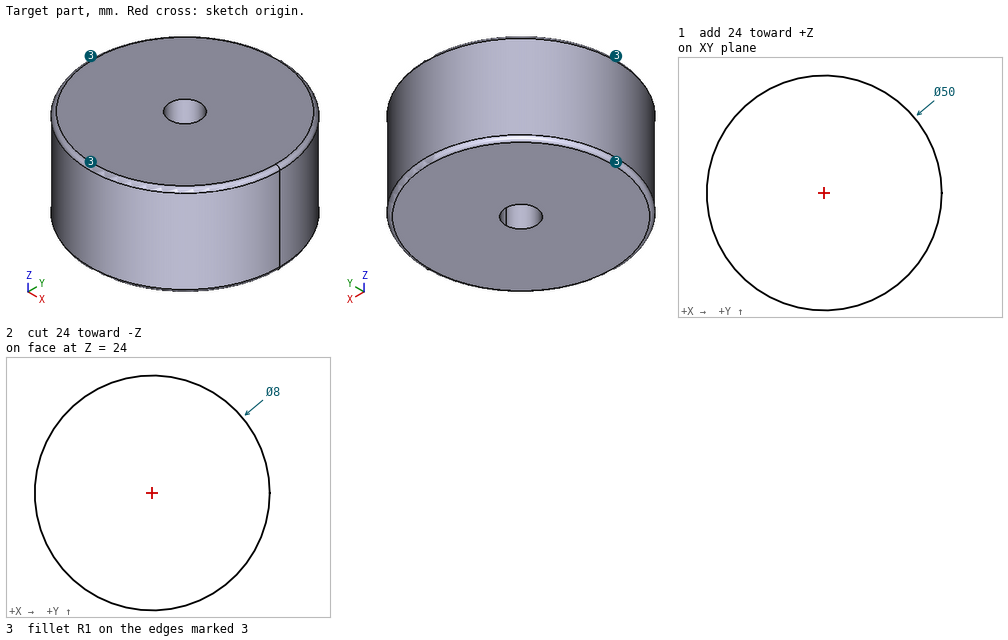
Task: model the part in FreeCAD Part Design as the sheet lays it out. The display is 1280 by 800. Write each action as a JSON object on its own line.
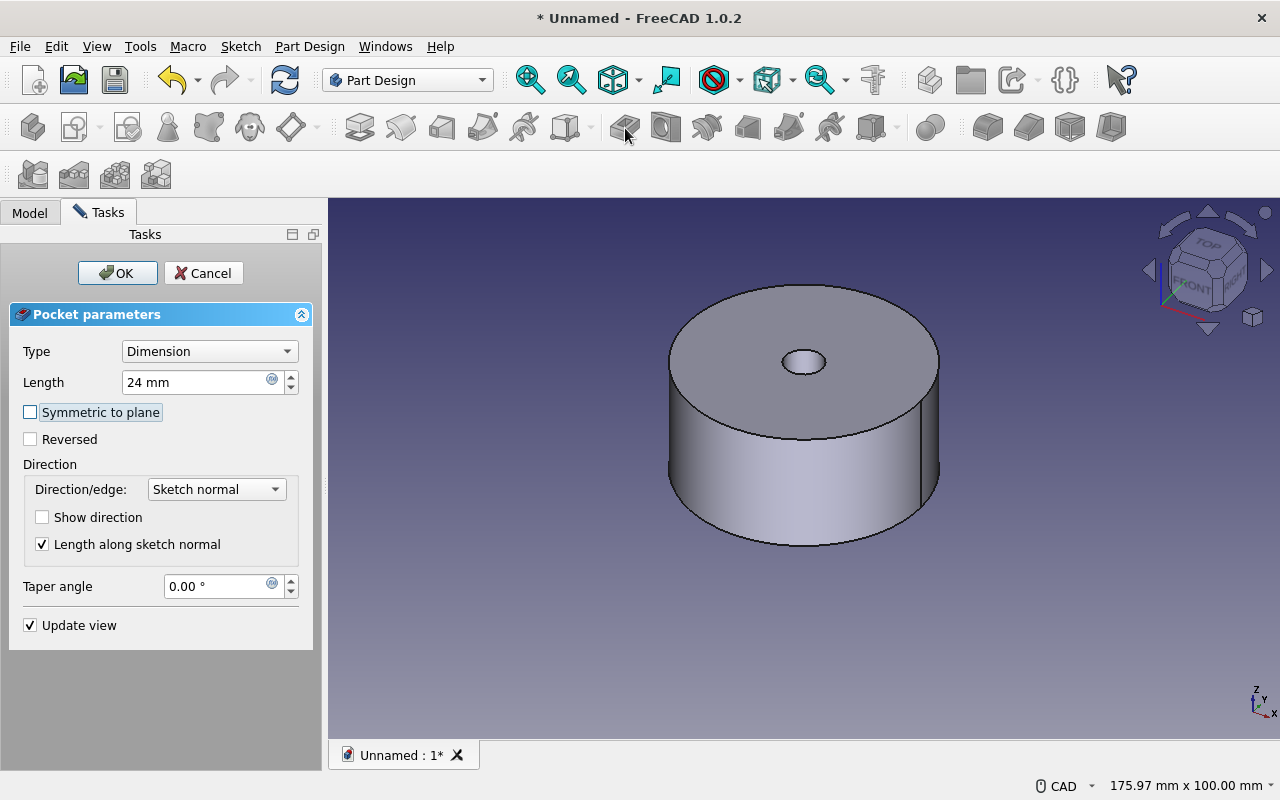
{"action": "left_click", "coordinate": [118, 273]}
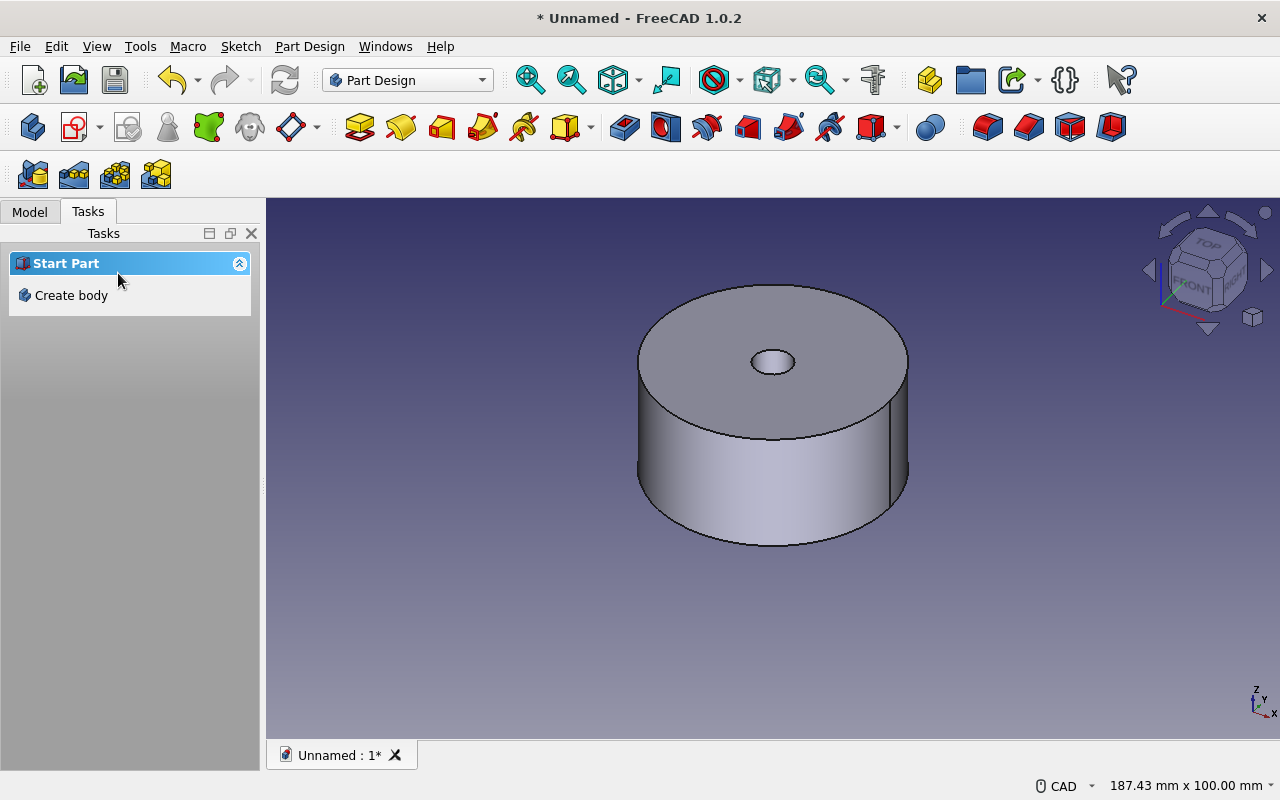
{"action": "left_click", "coordinate": [638, 369]}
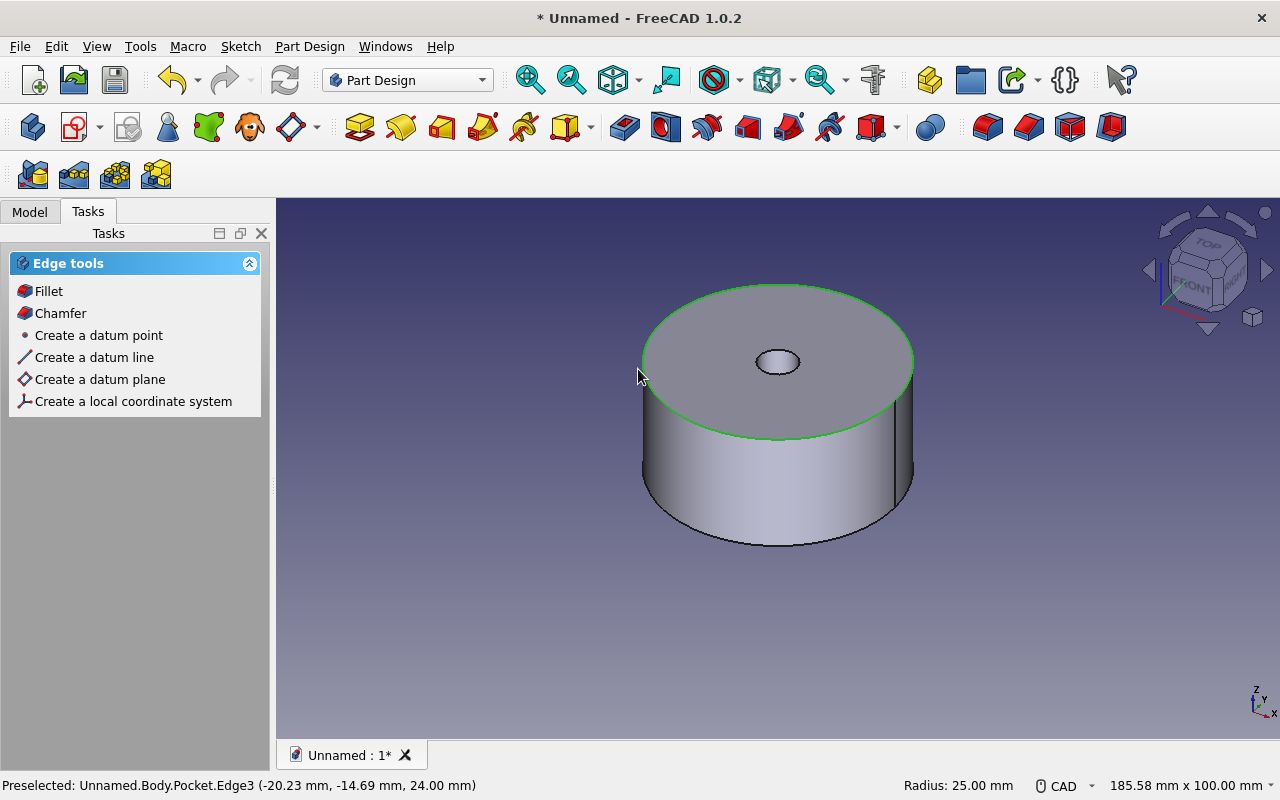
{"action": "key", "text": "0"}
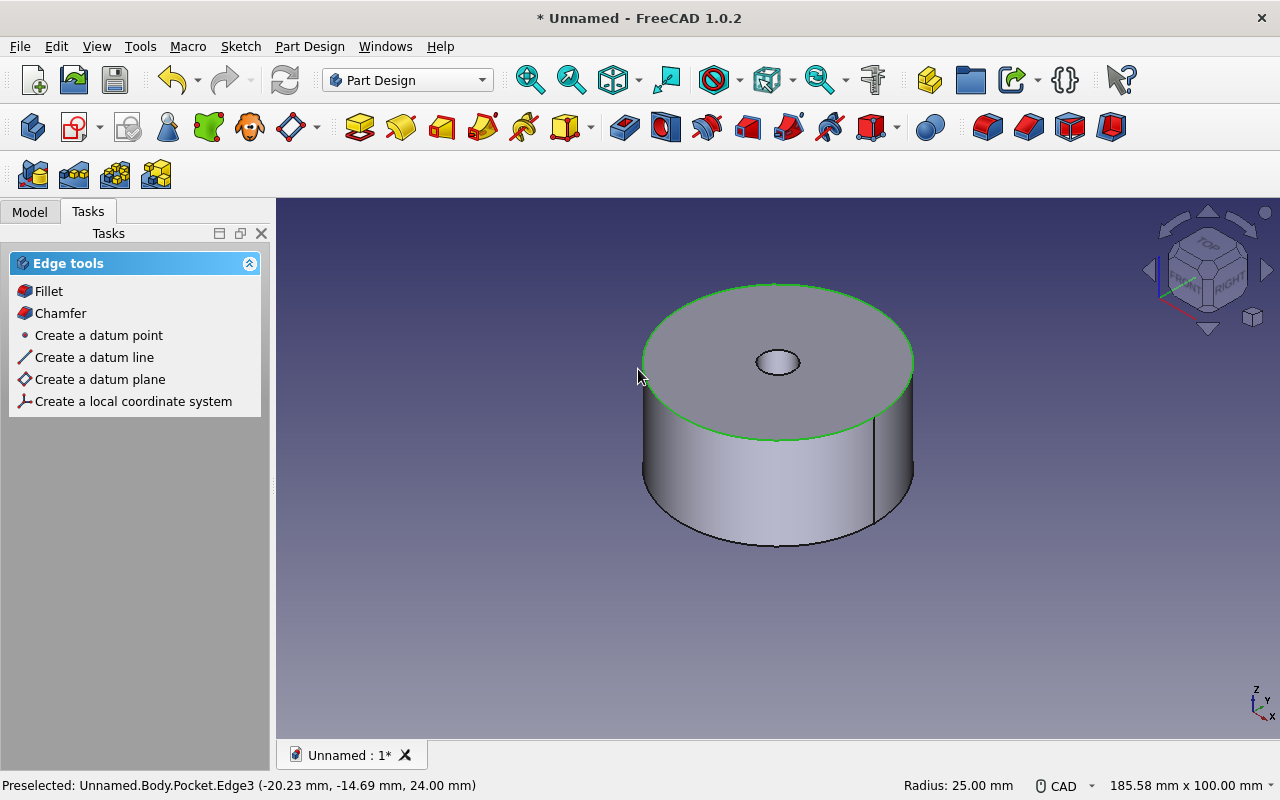
{"action": "key", "text": "2"}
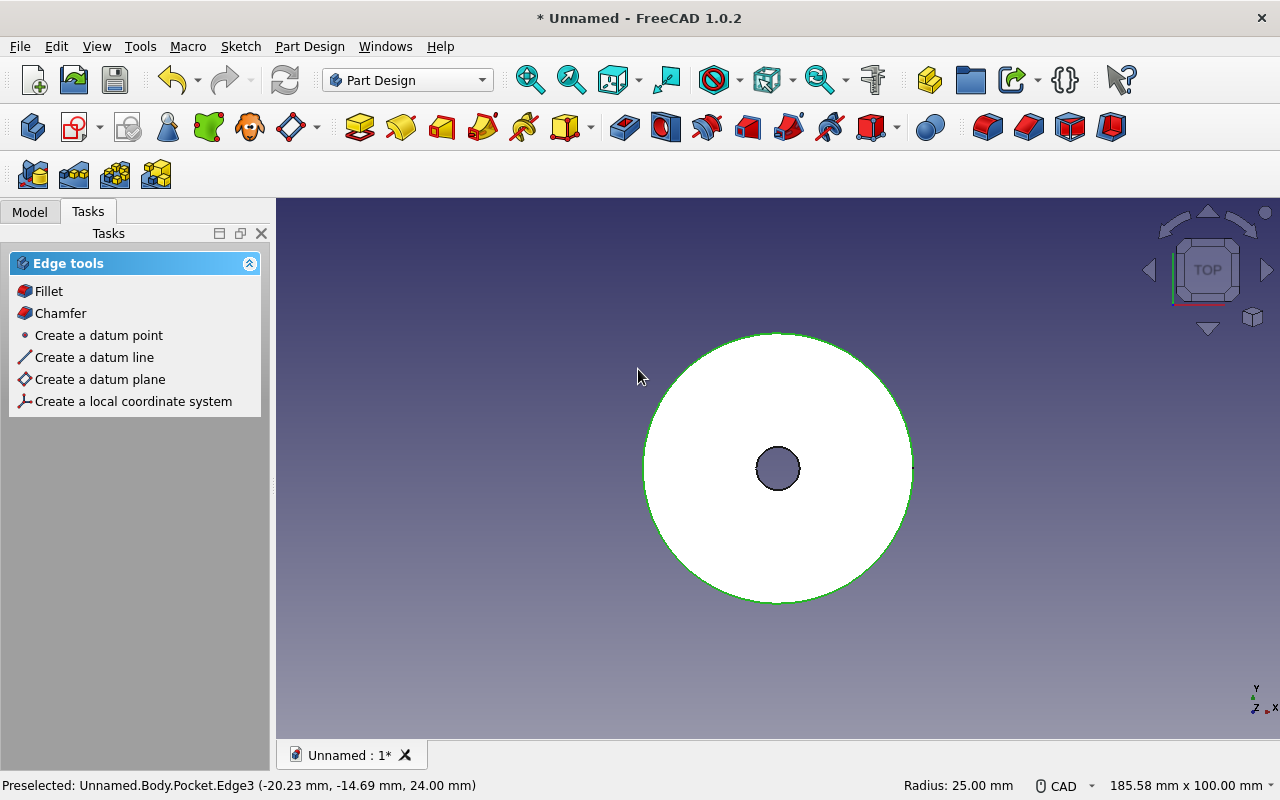
{"action": "key", "text": "1"}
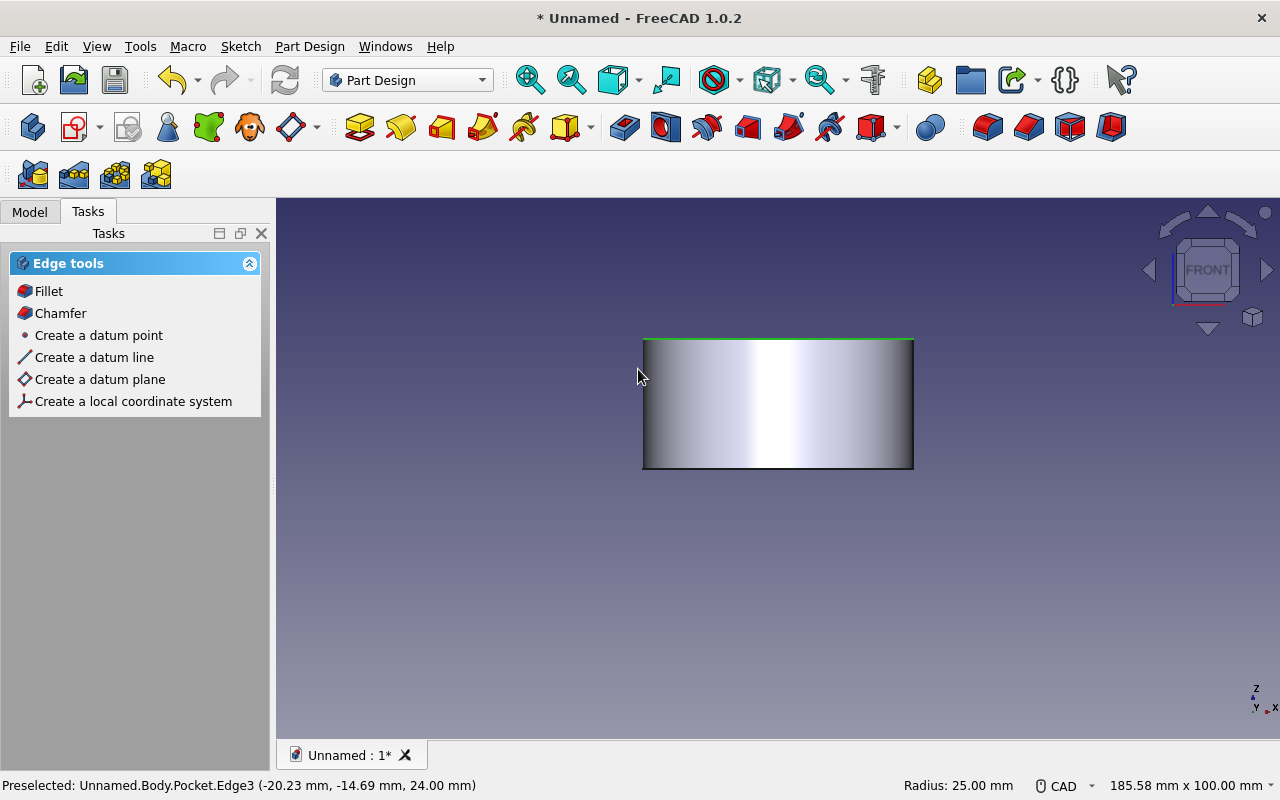
{"action": "left_click", "coordinate": [531, 80]}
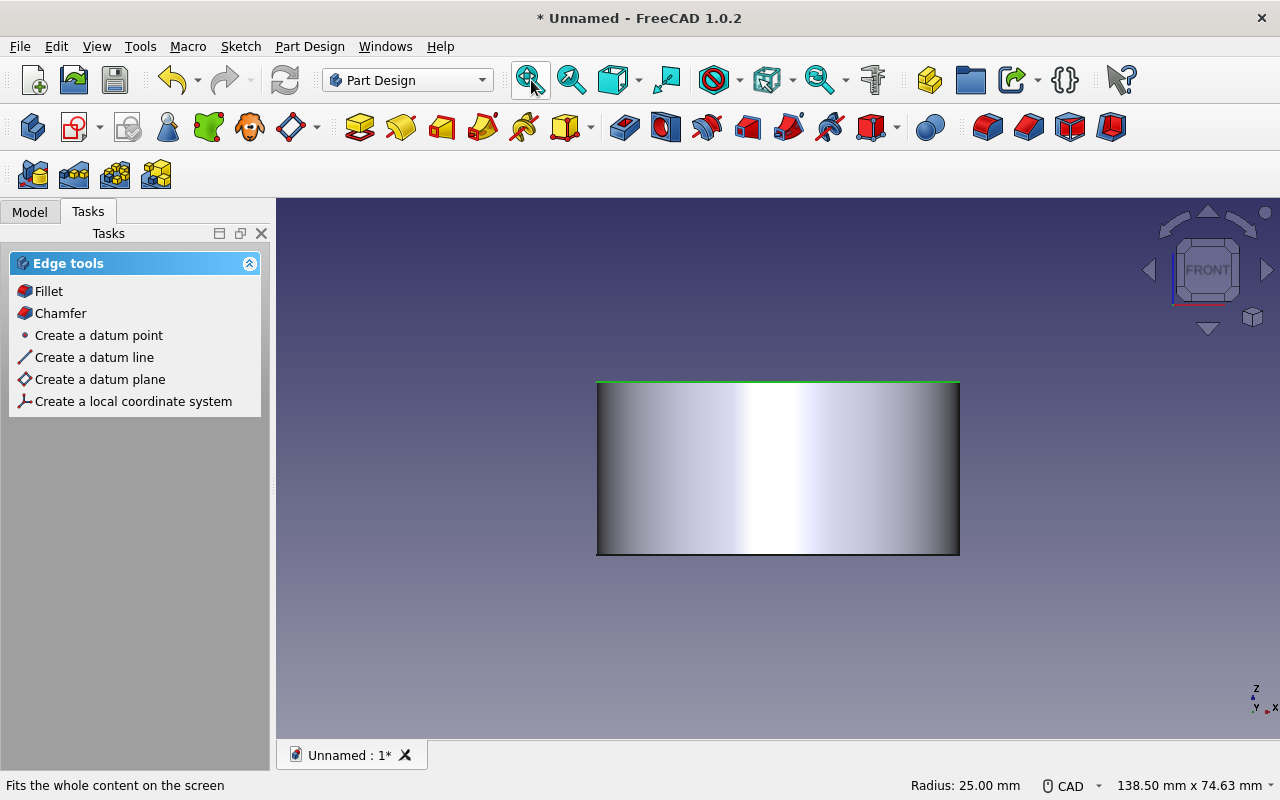
{"action": "left_click", "coordinate": [631, 554], "text": "ctrl"}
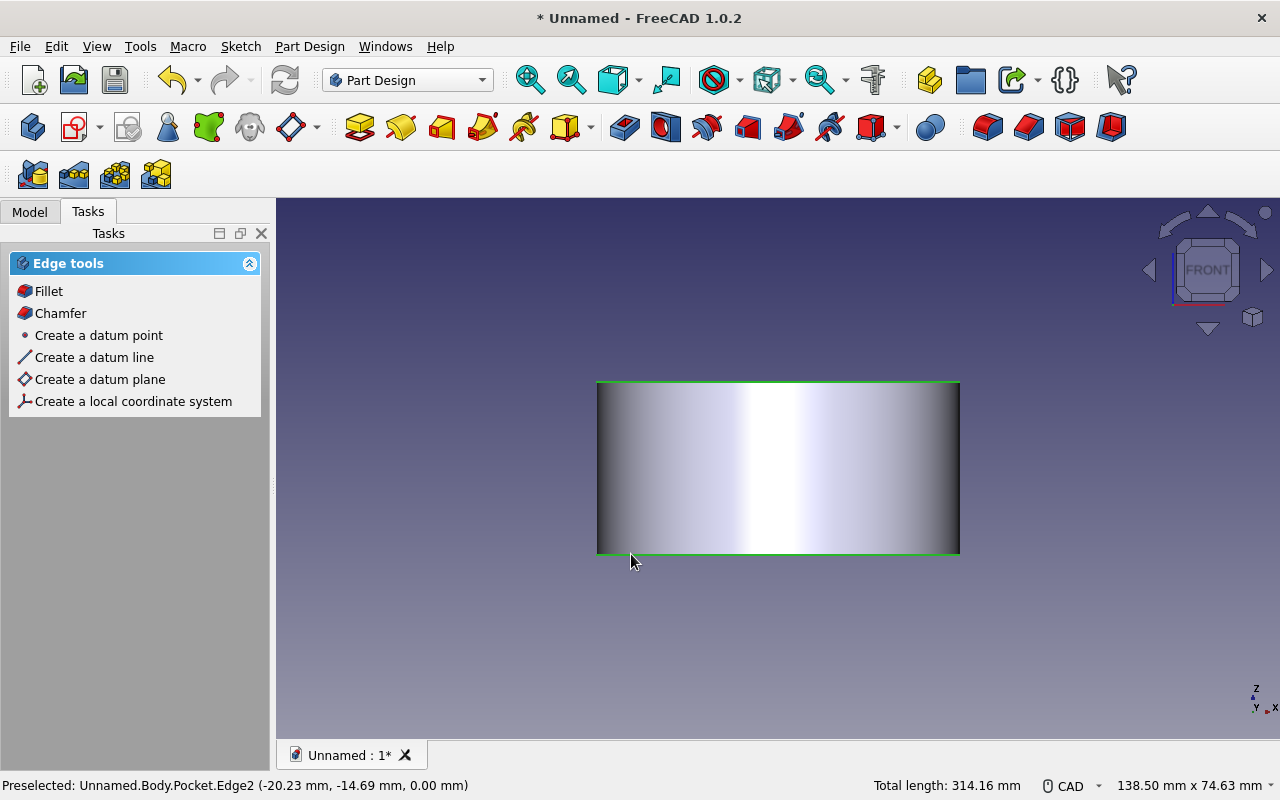
{"action": "left_click", "coordinate": [988, 128]}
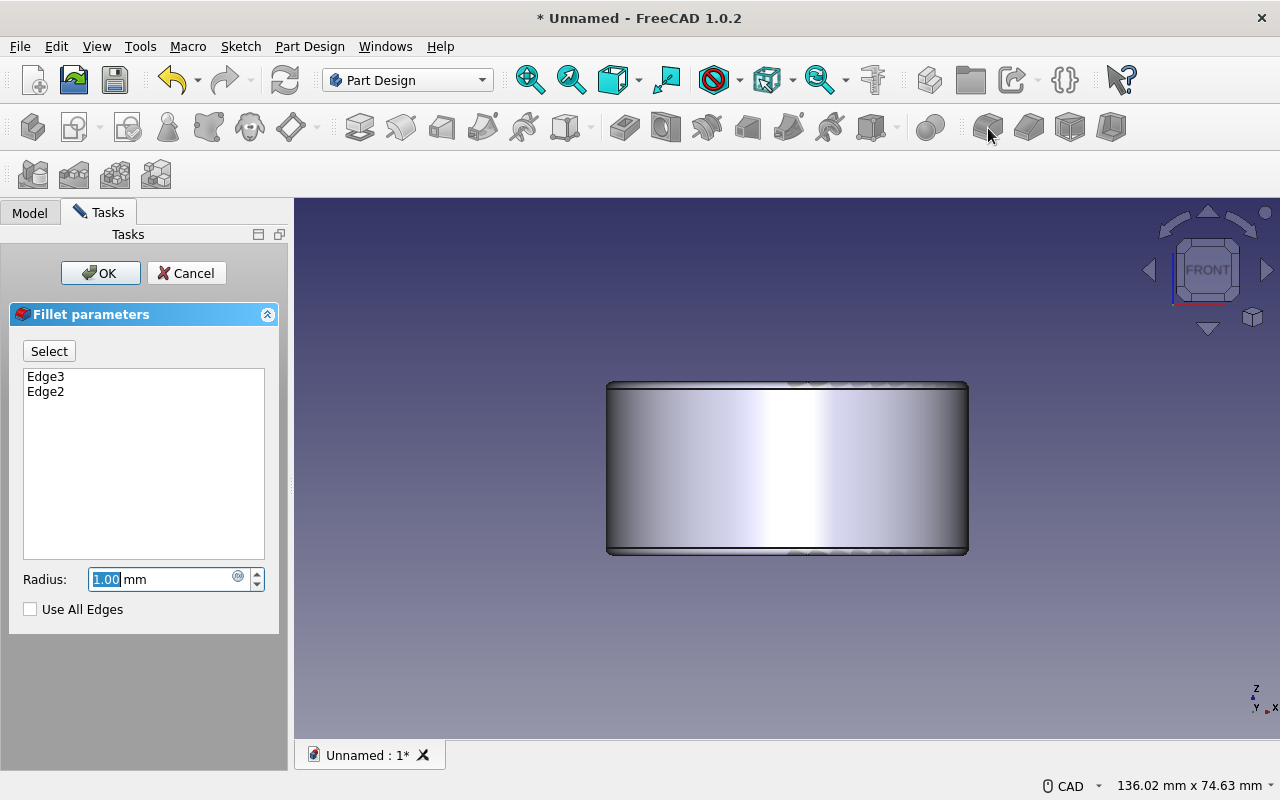
{"action": "type", "text": "1"}
{"action": "key", "text": "Tab"}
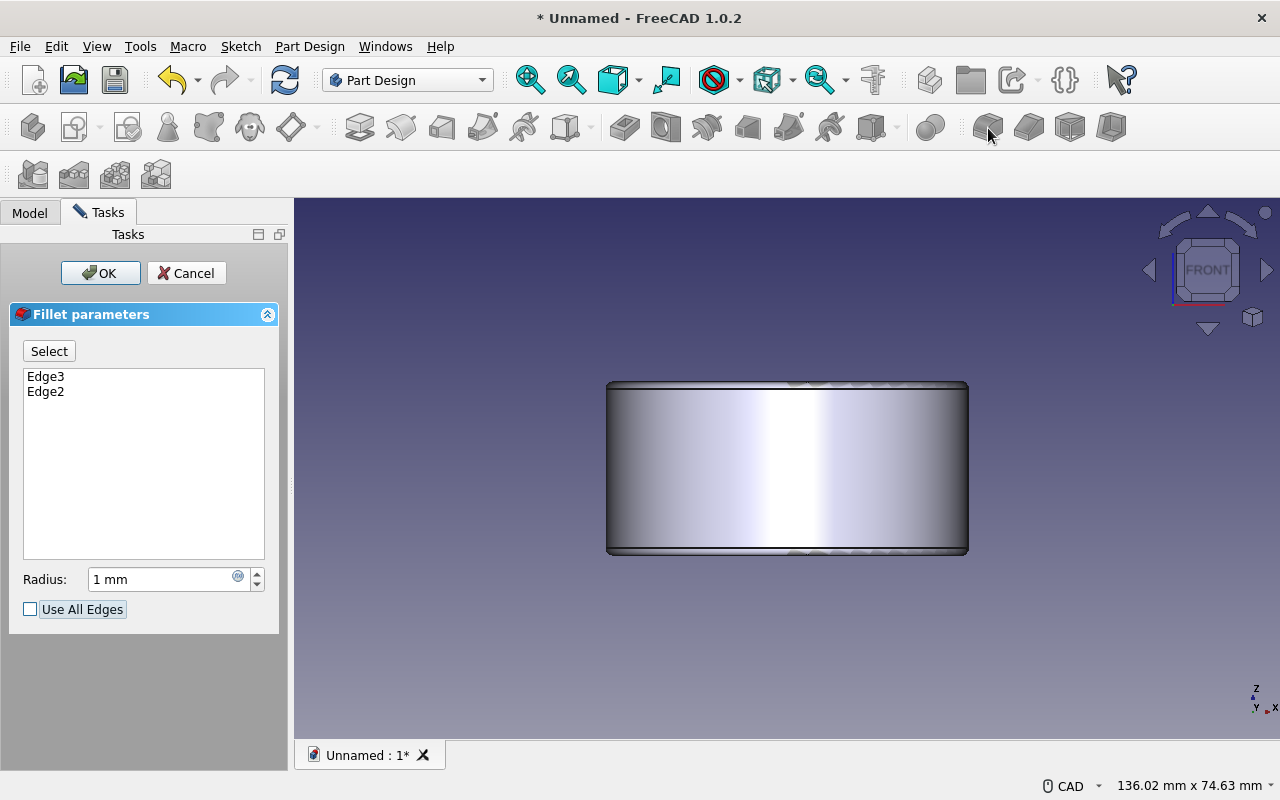
{"action": "left_click", "coordinate": [101, 273]}